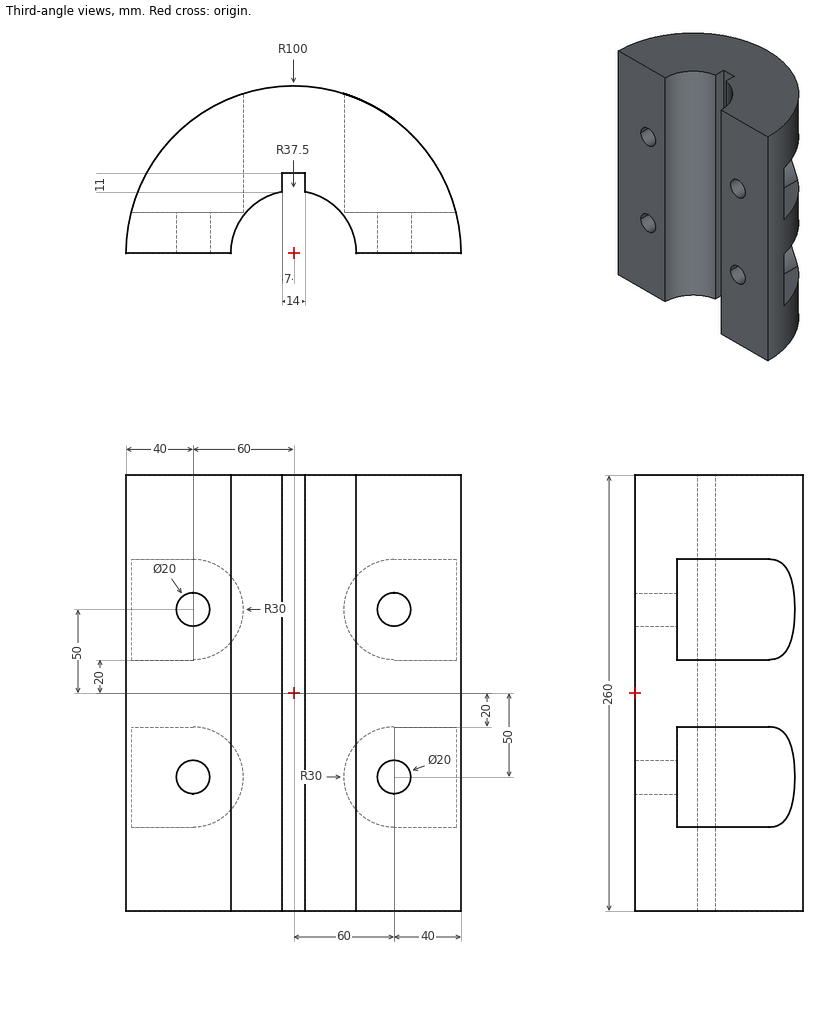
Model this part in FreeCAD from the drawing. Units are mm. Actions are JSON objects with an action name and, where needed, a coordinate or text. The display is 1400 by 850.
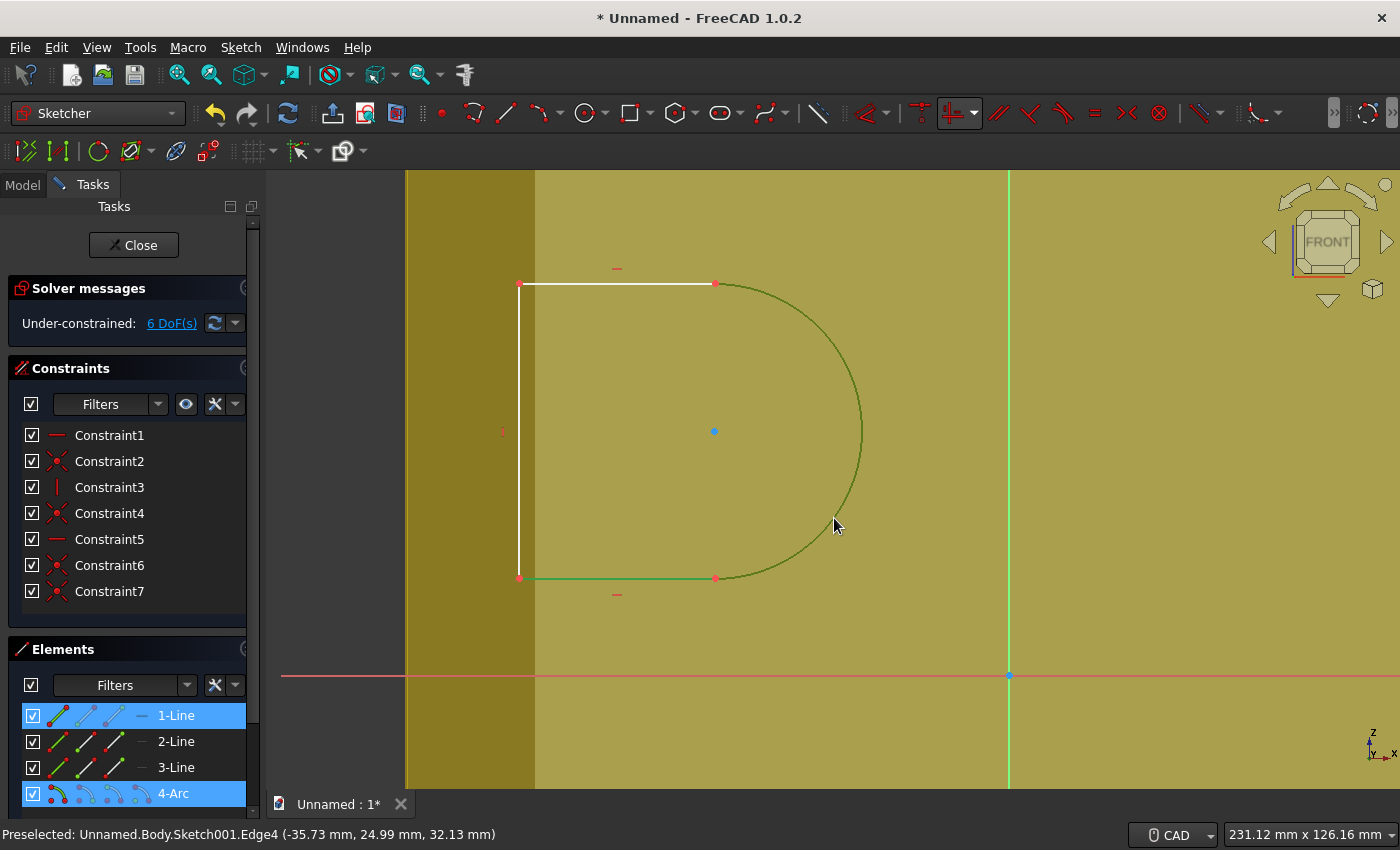
{"action": "left_click", "coordinate": [1064, 114]}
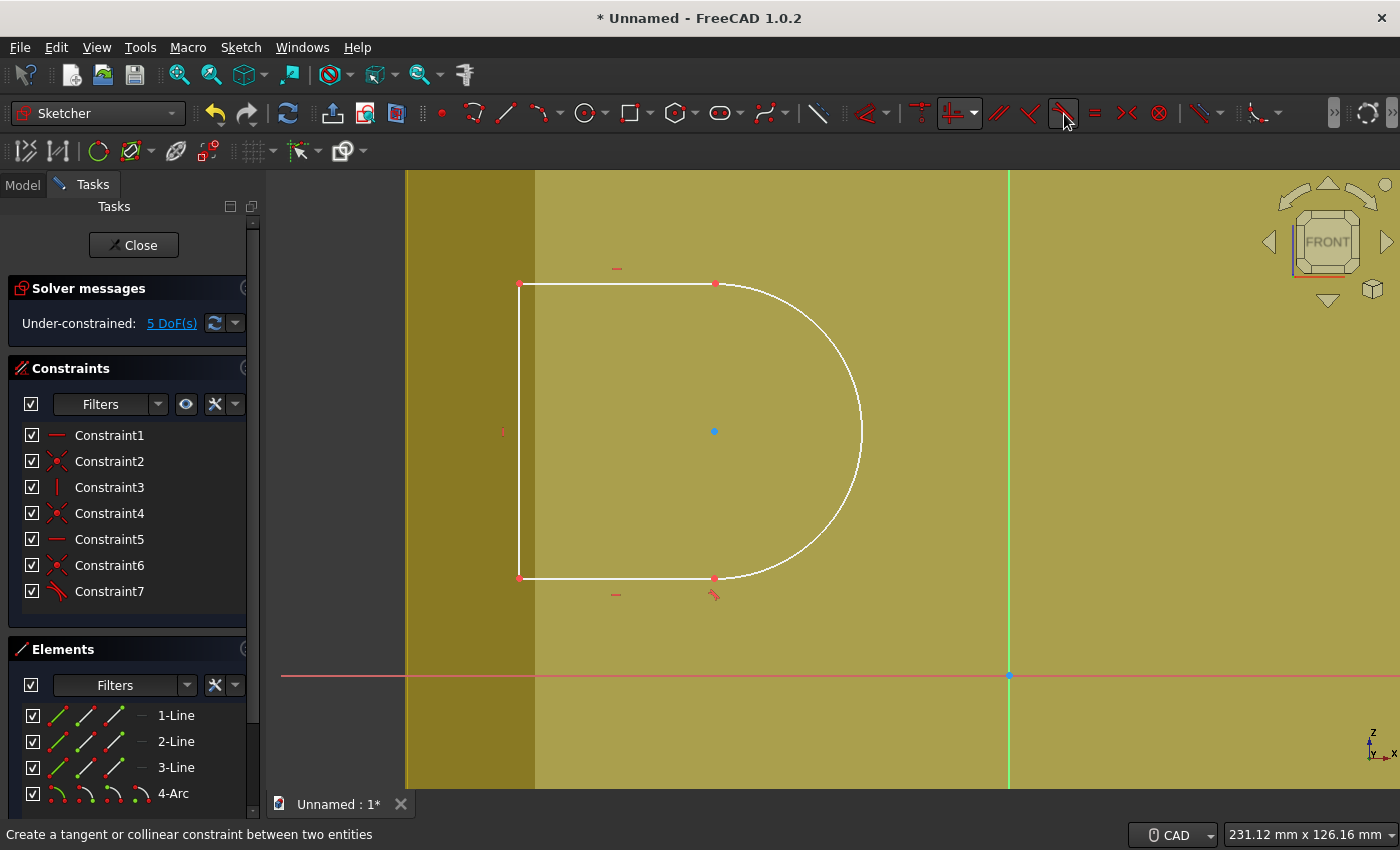
{"action": "left_click", "coordinate": [578, 284]}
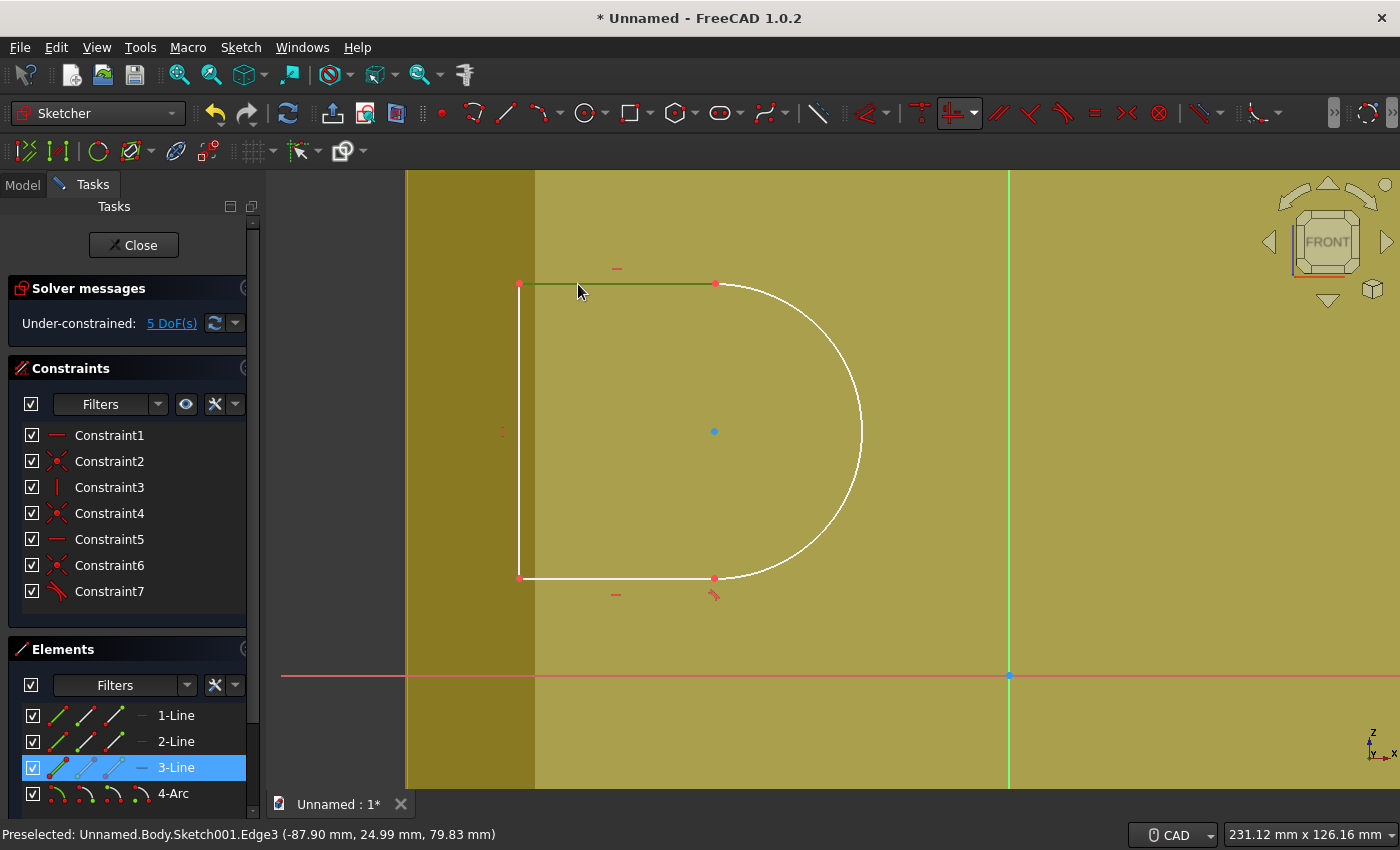
{"action": "left_click", "coordinate": [834, 518]}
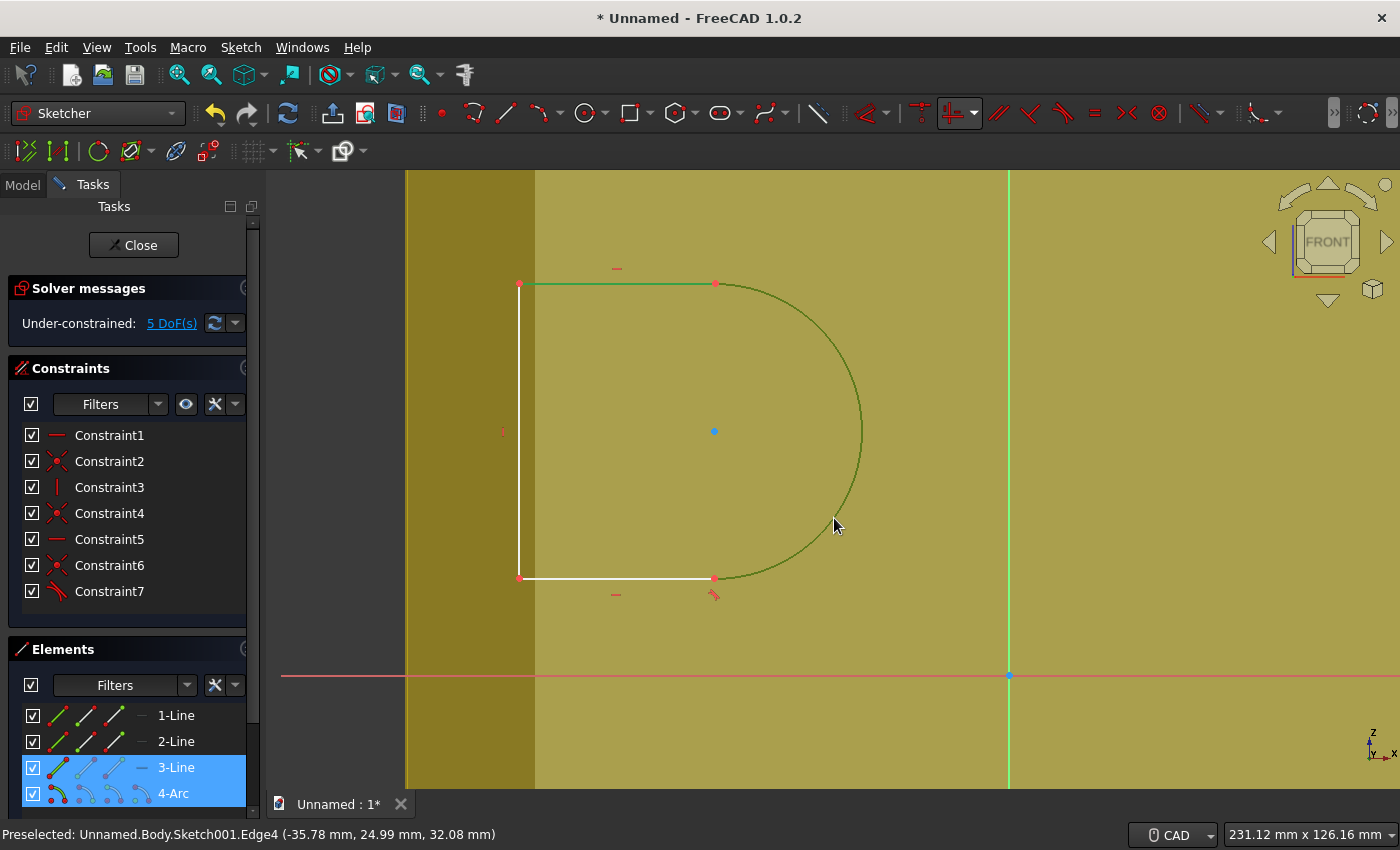
{"action": "left_click", "coordinate": [1064, 114]}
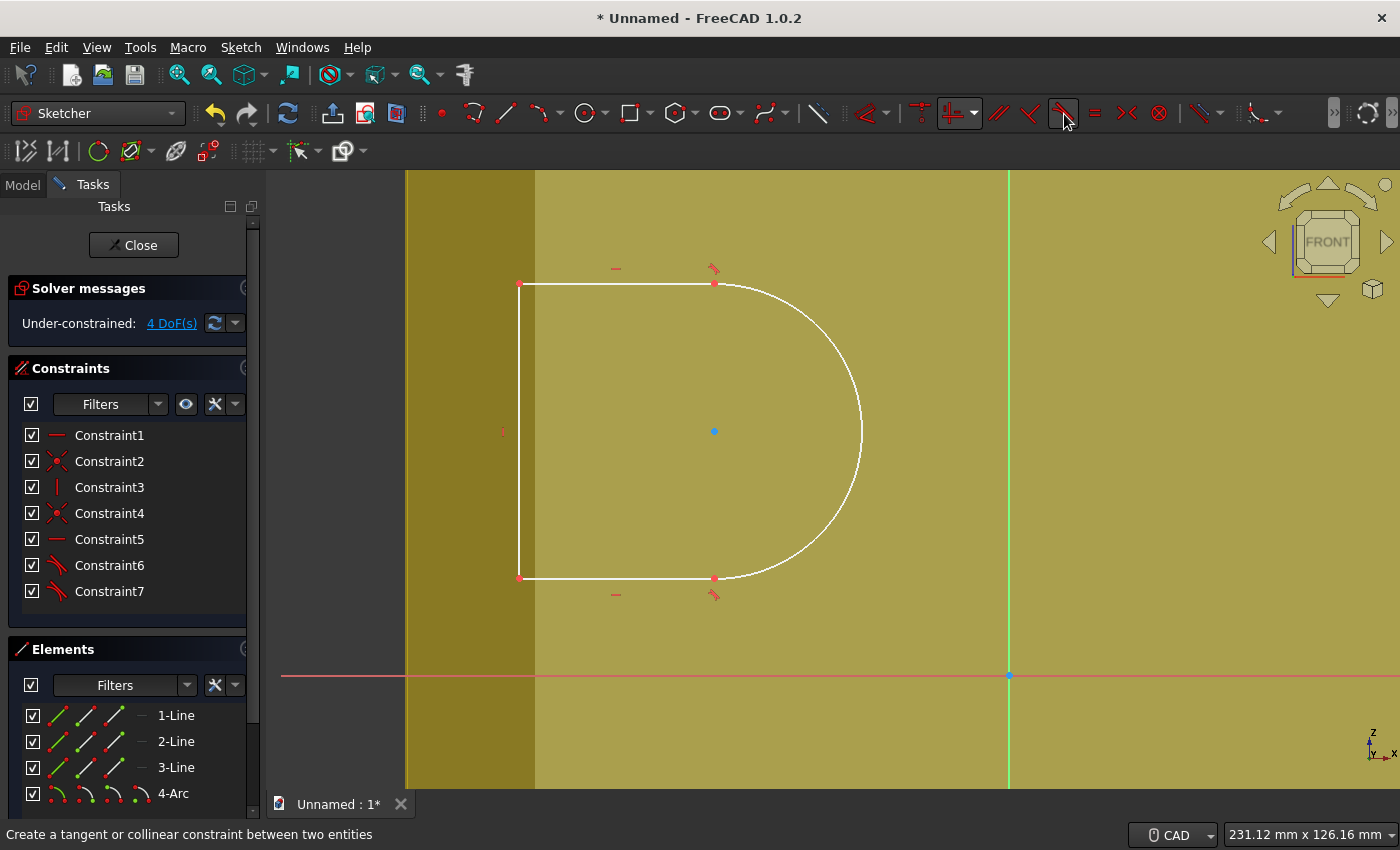
{"action": "left_click", "coordinate": [866, 114]}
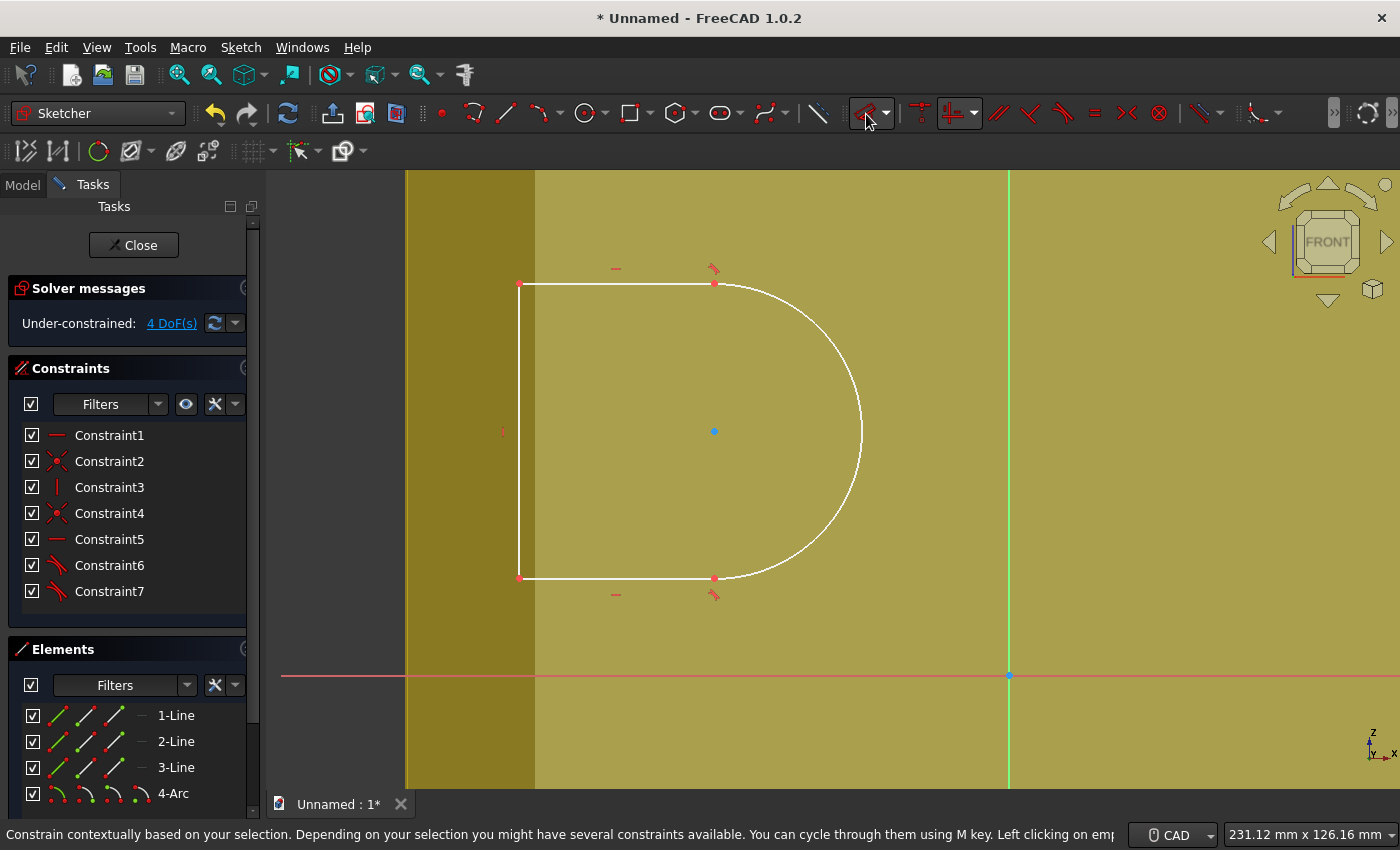
{"action": "left_click", "coordinate": [834, 518]}
{"action": "left_click", "coordinate": [860, 537]}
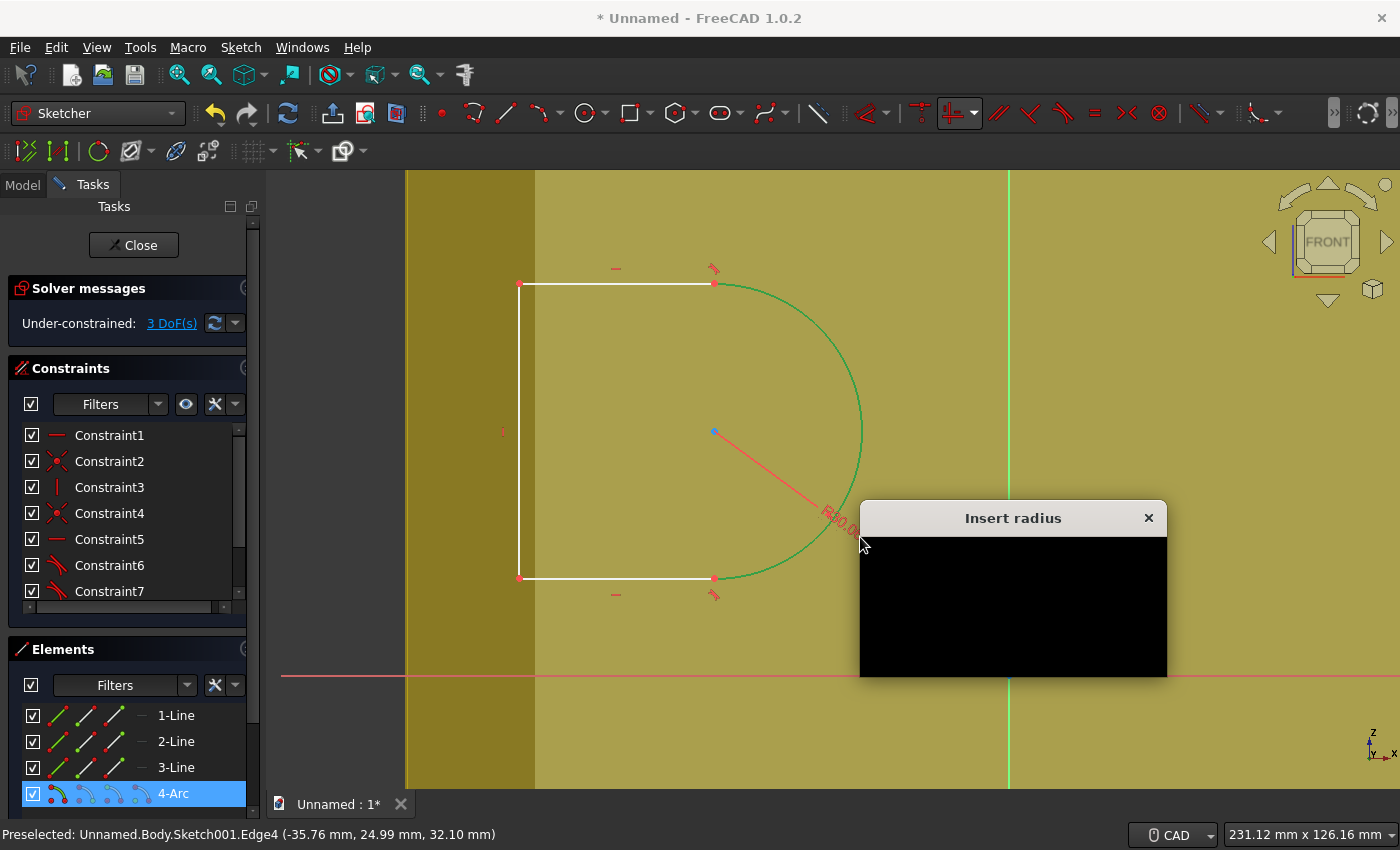
{"action": "type", "text": "30"}
{"action": "key", "text": "Return"}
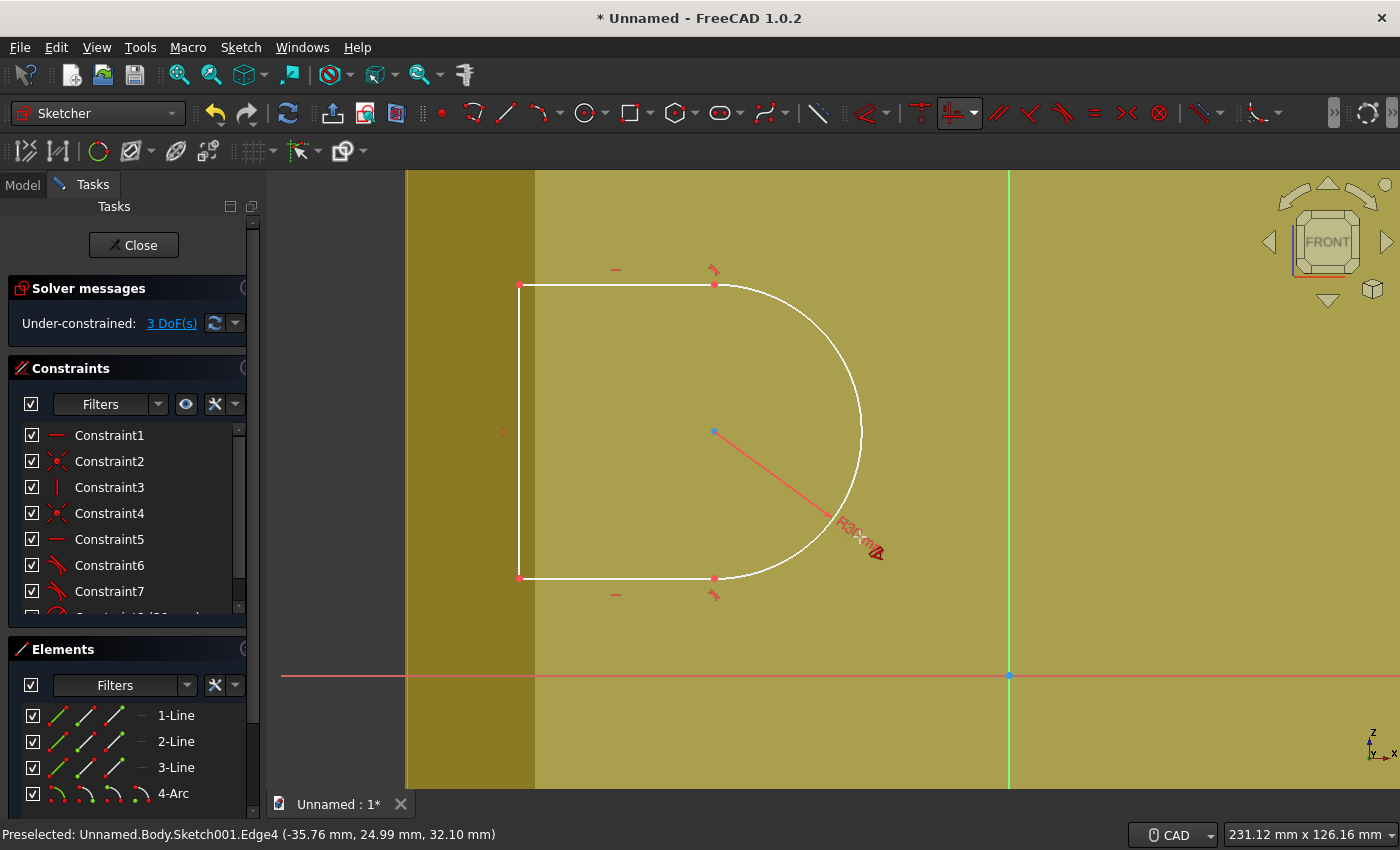
{"action": "left_click", "coordinate": [656, 579]}
{"action": "left_click", "coordinate": [617, 613]}